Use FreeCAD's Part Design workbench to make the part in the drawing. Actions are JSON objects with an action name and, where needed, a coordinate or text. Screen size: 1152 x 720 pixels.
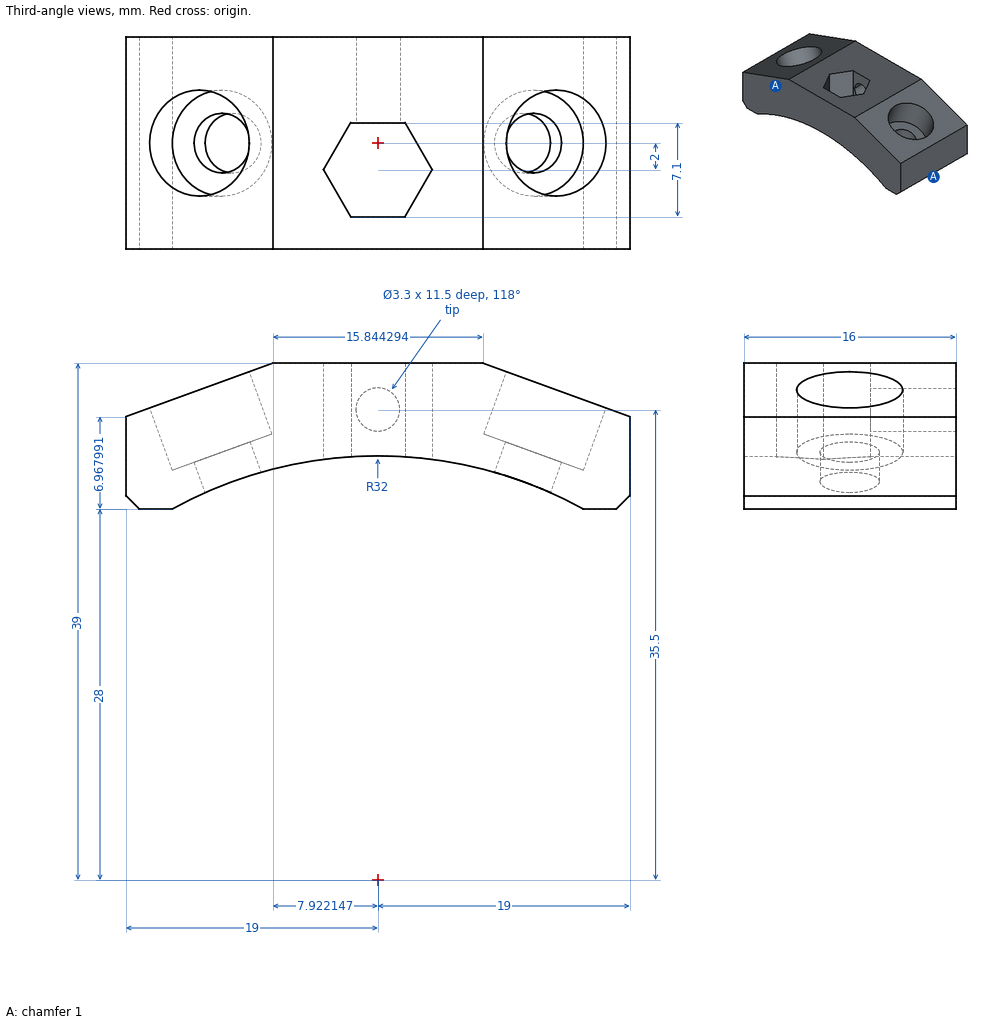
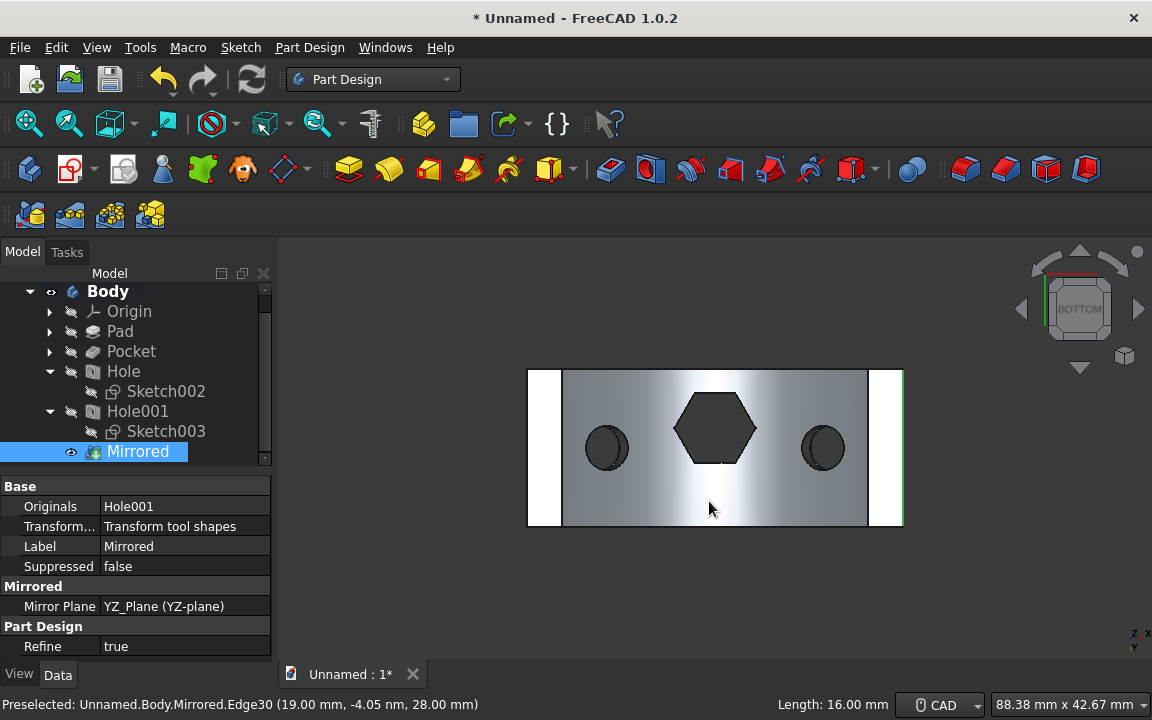
{"action": "left_click", "coordinate": [30, 124]}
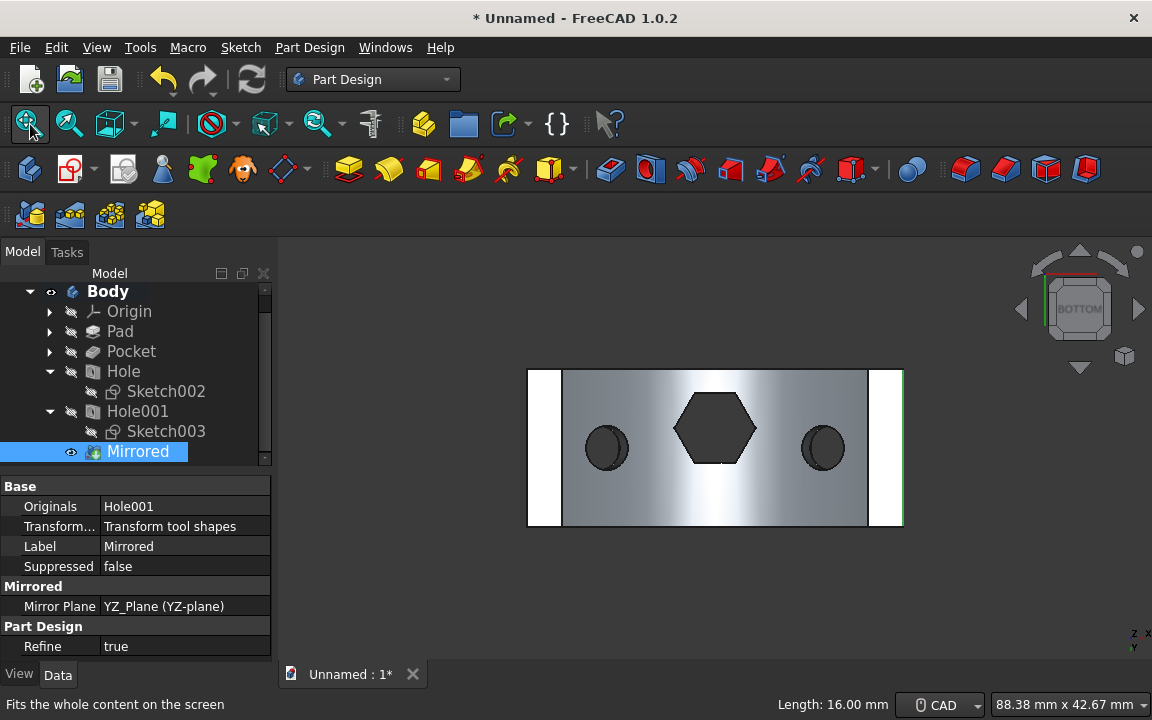
{"action": "left_click", "coordinate": [527, 447], "text": "ctrl"}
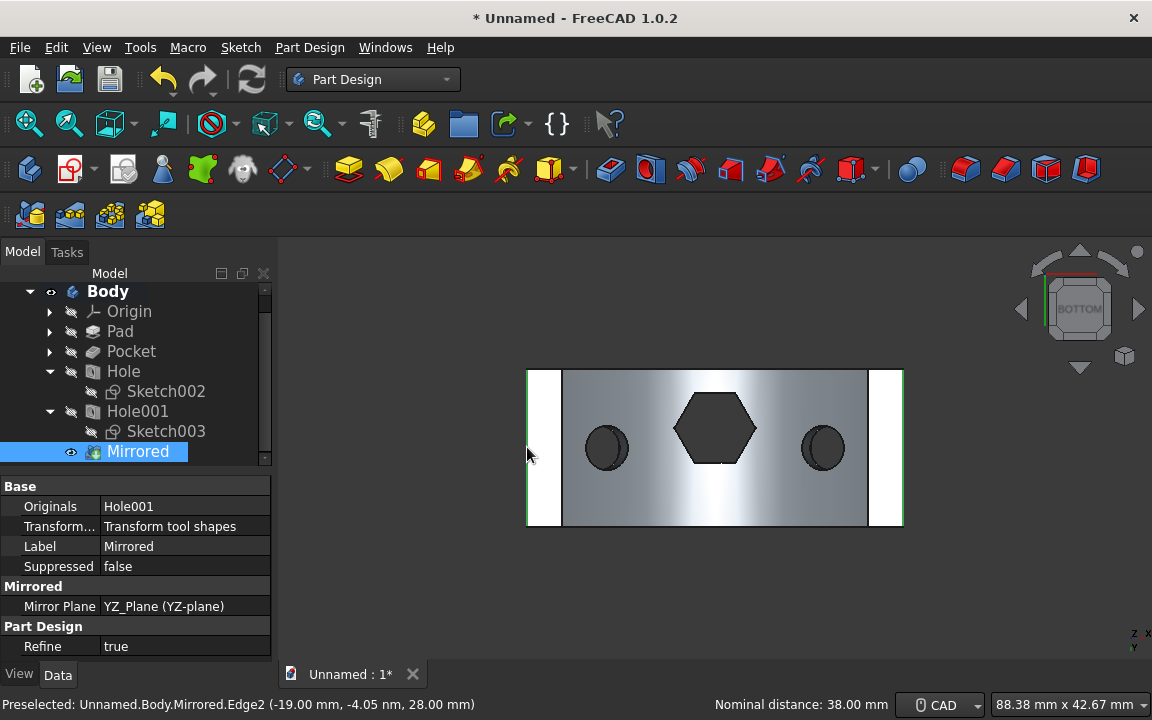
{"action": "left_click", "coordinate": [1006, 170]}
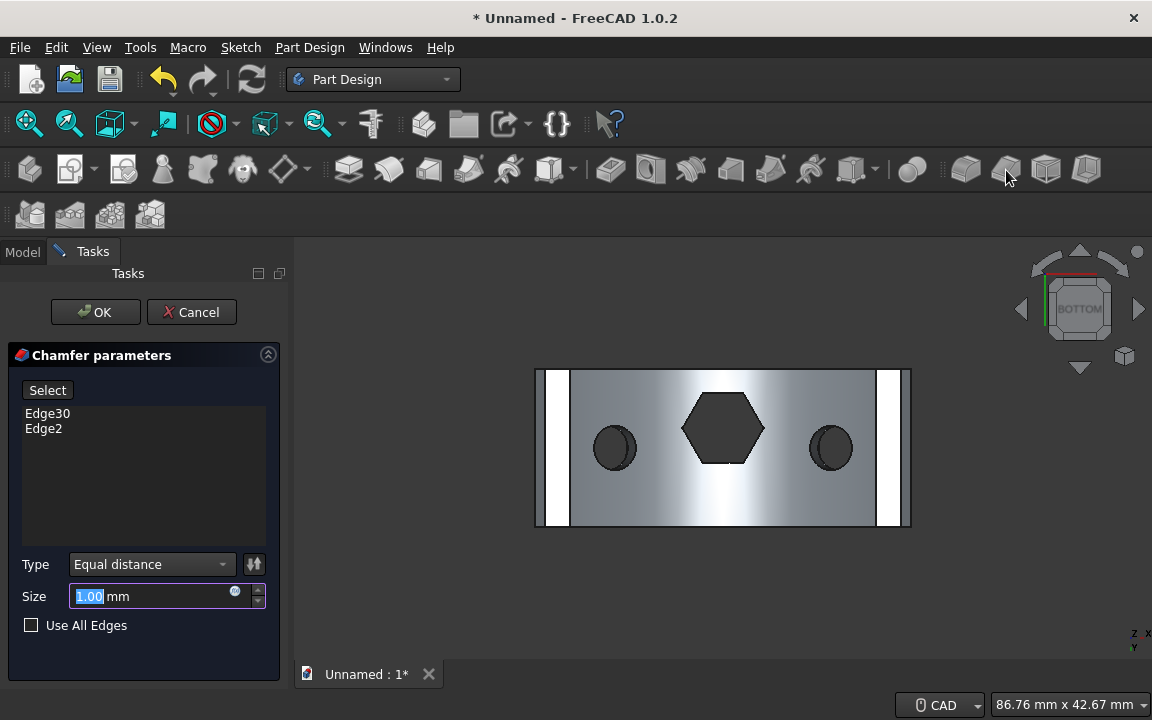
{"action": "type", "text": "1"}
{"action": "key", "text": "Tab"}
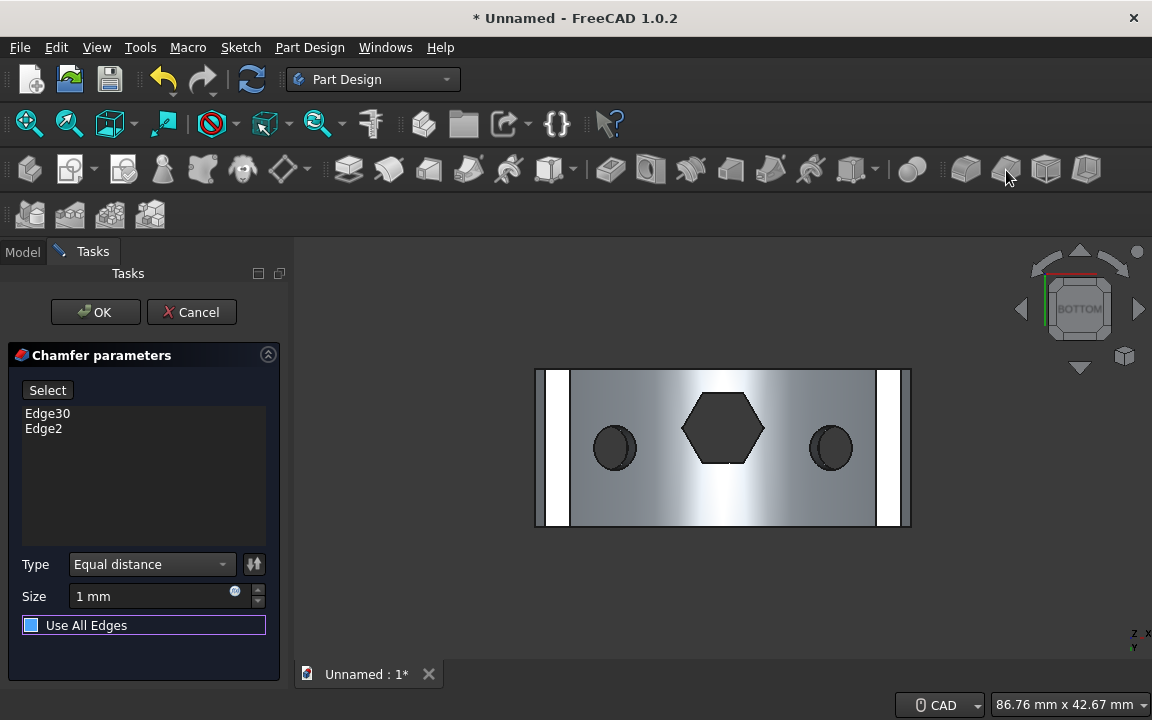
{"action": "left_click", "coordinate": [96, 312]}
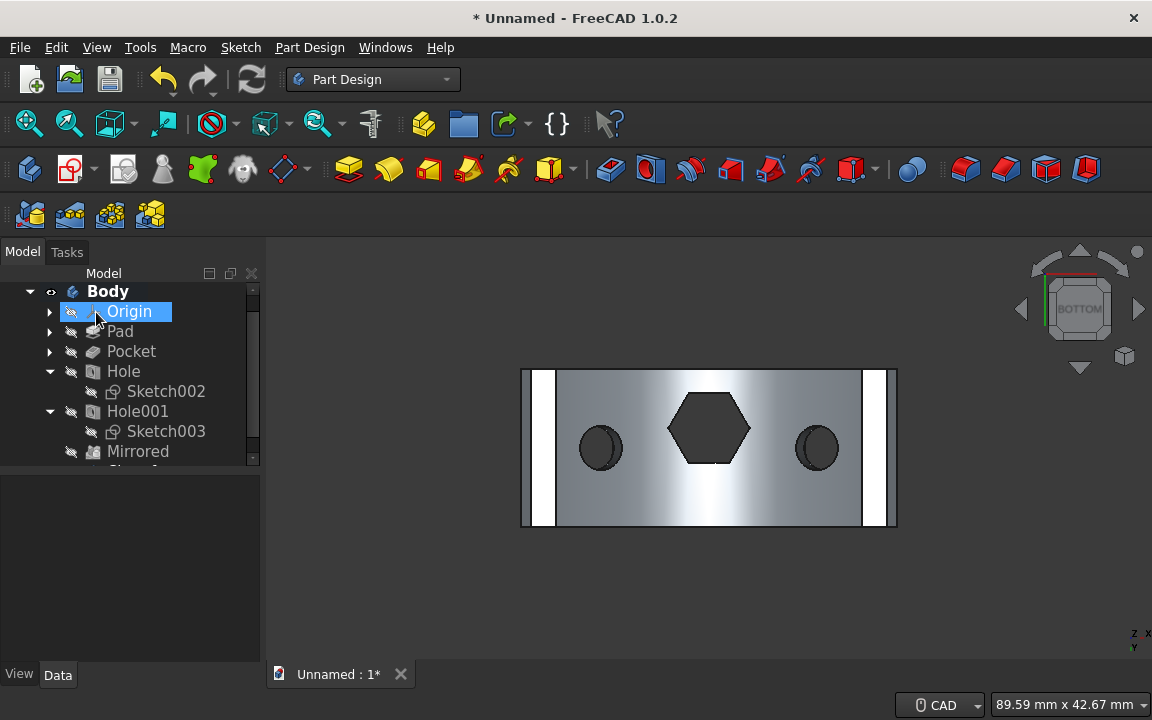
{"action": "key", "text": "0"}